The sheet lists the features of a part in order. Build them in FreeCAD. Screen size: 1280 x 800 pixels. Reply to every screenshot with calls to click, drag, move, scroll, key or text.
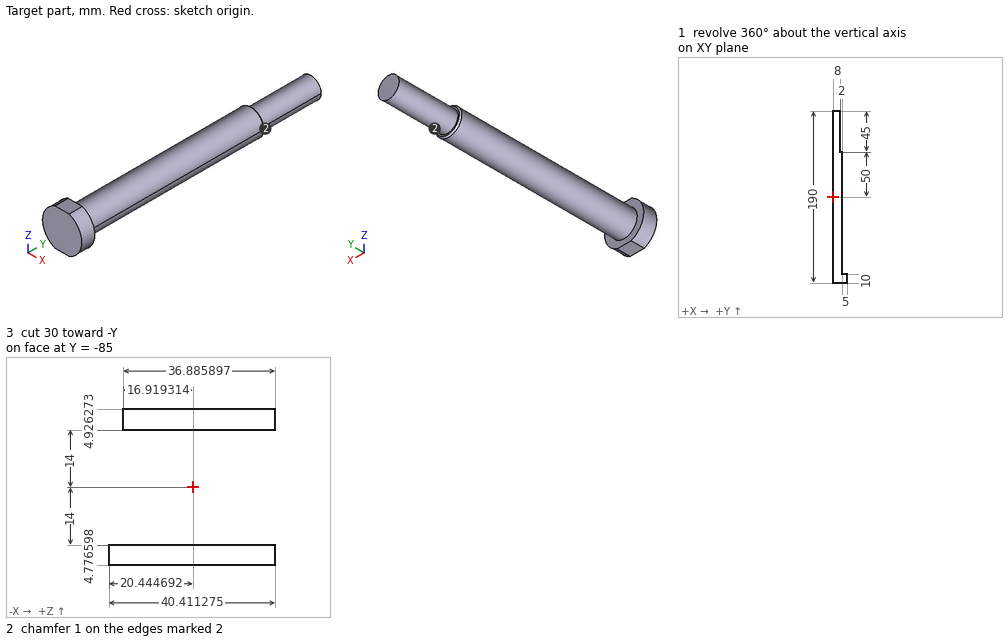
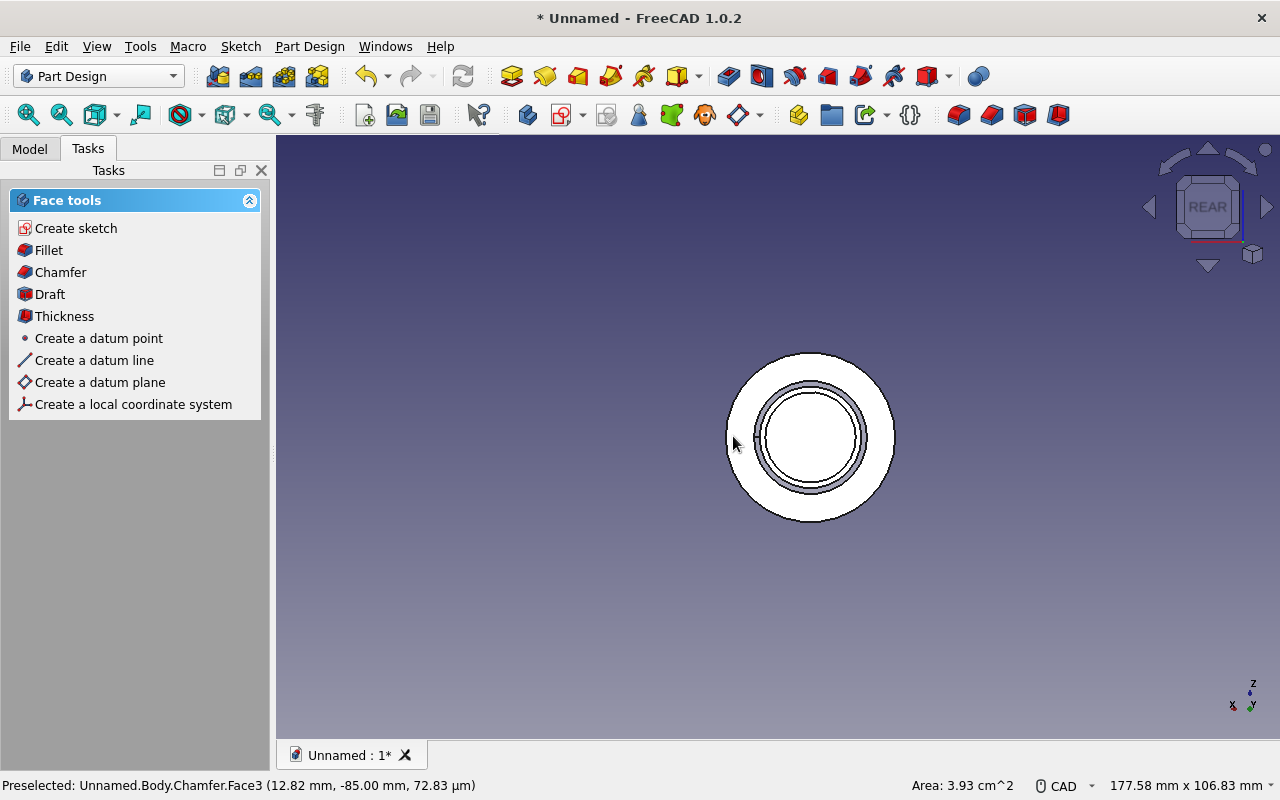
click(560, 116)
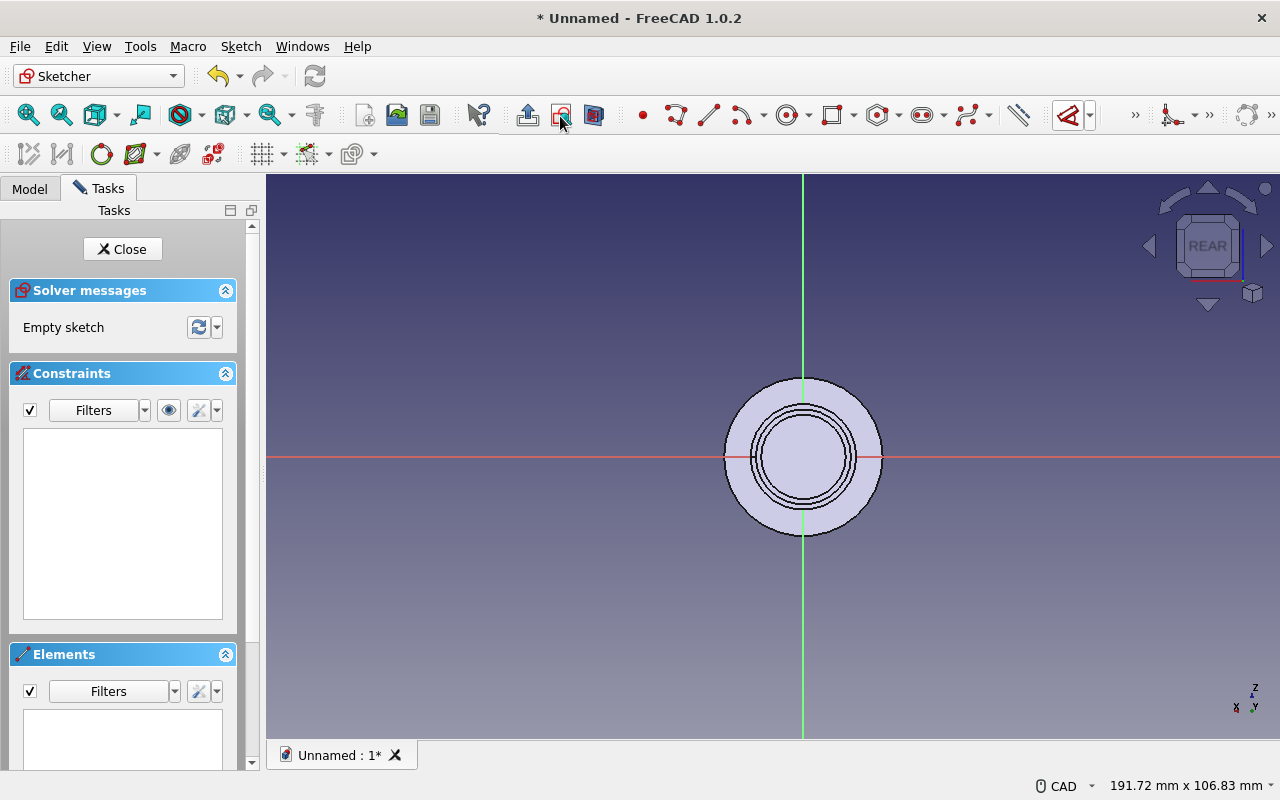
scroll(921, 456, up, 3)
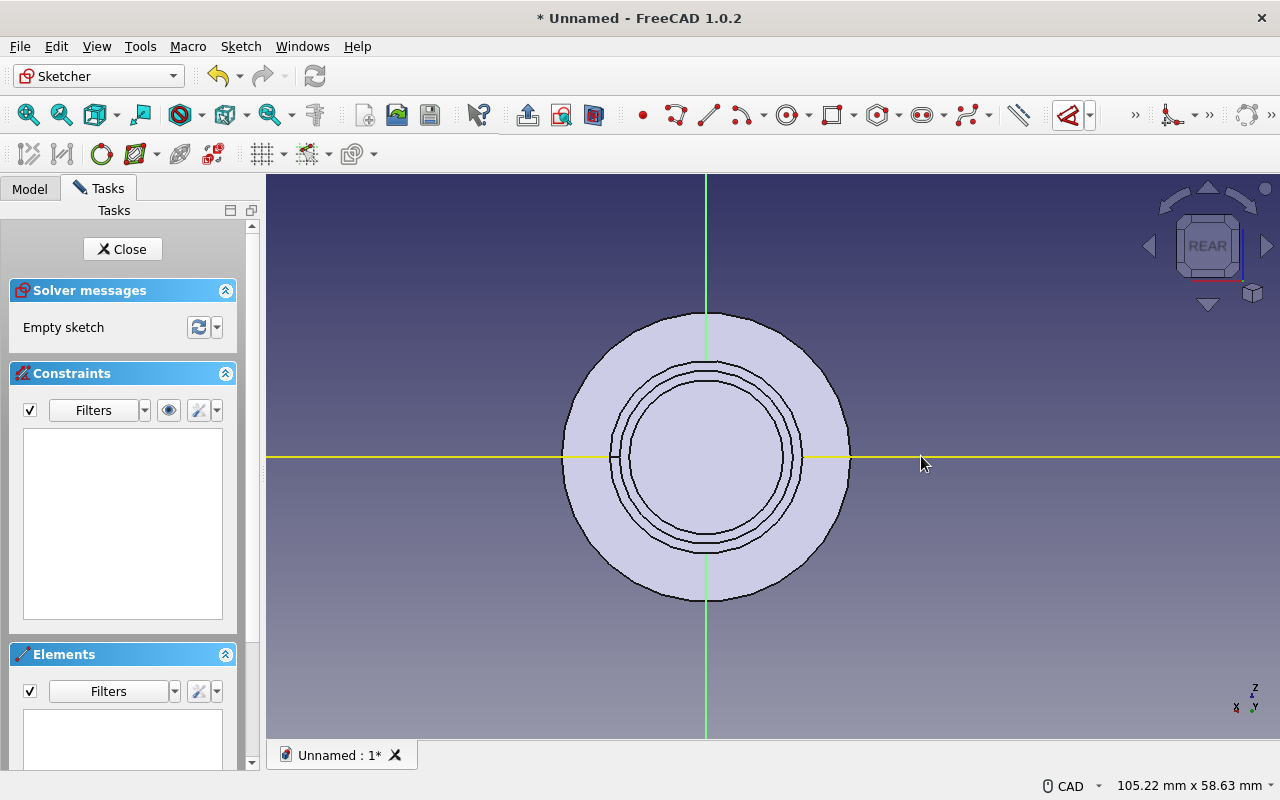
click(832, 116)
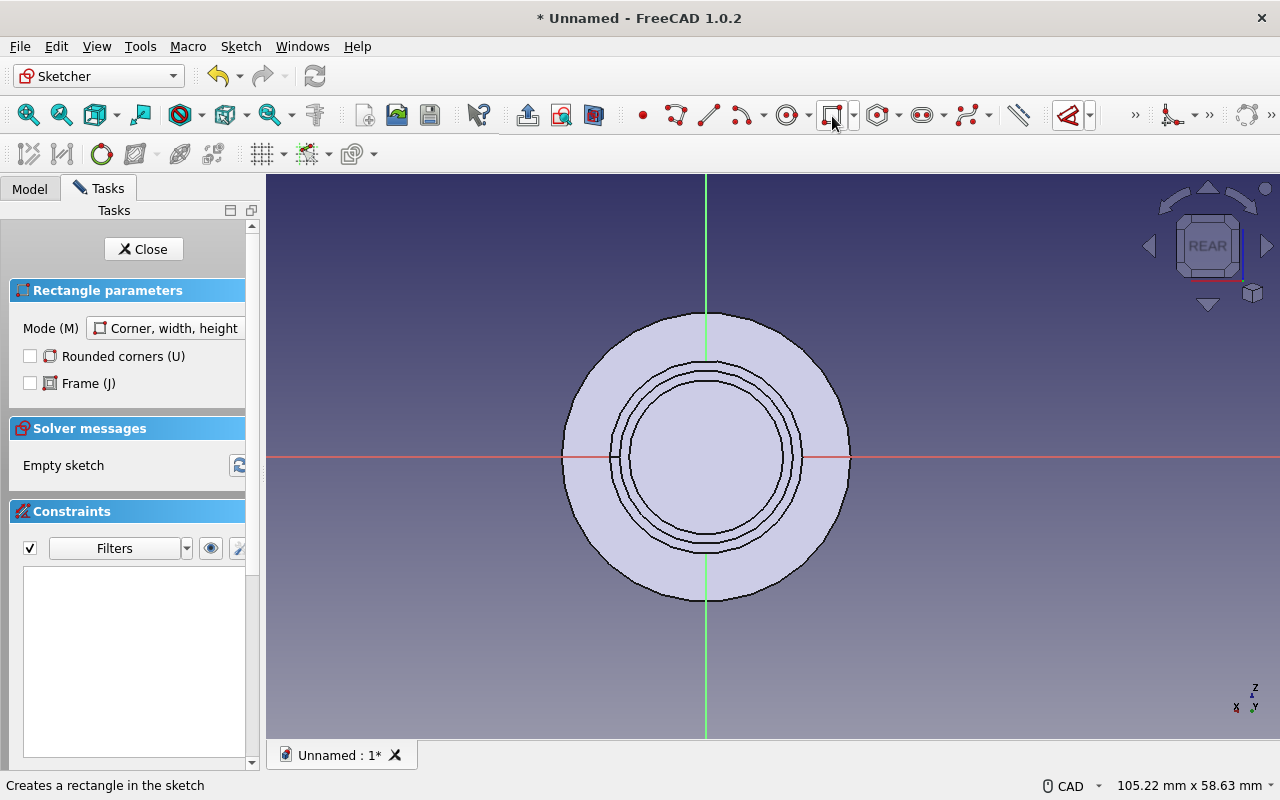
click(543, 275)
click(899, 322)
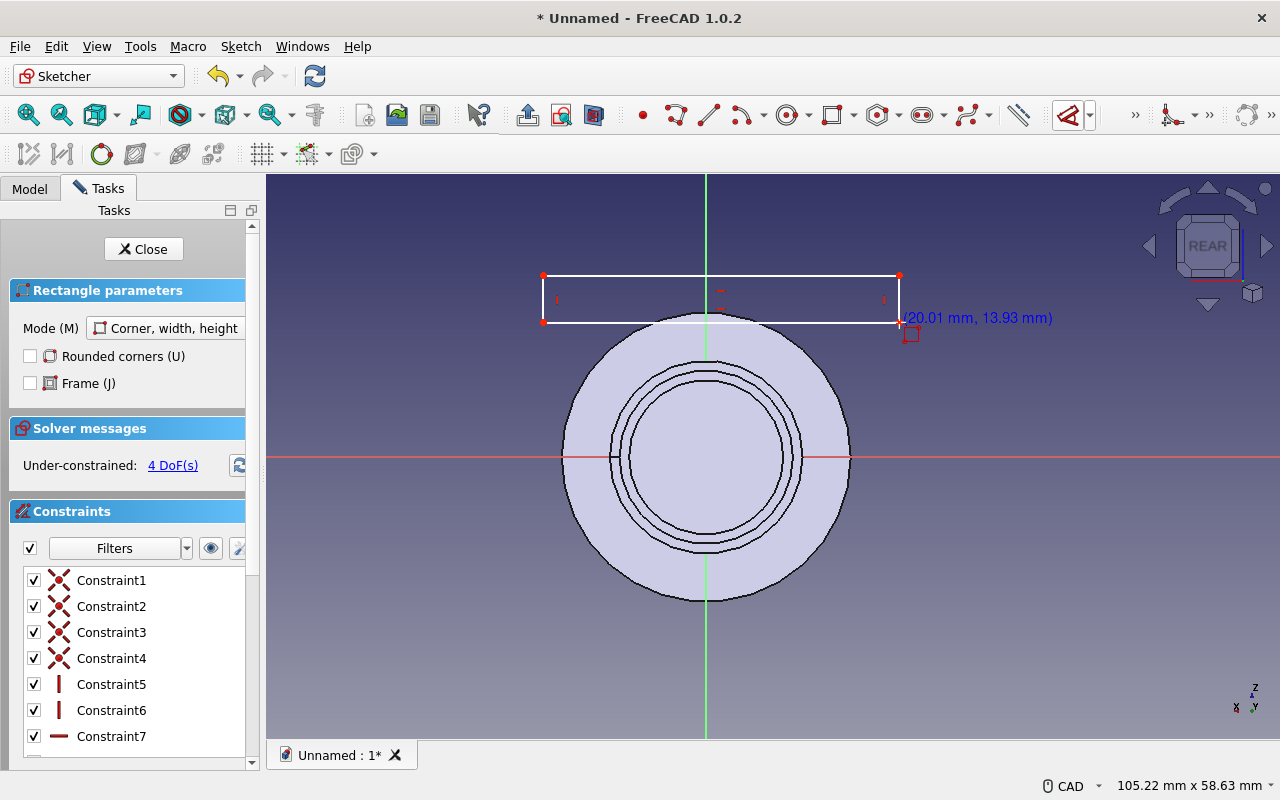
click(509, 592)
click(899, 638)
key(Escape)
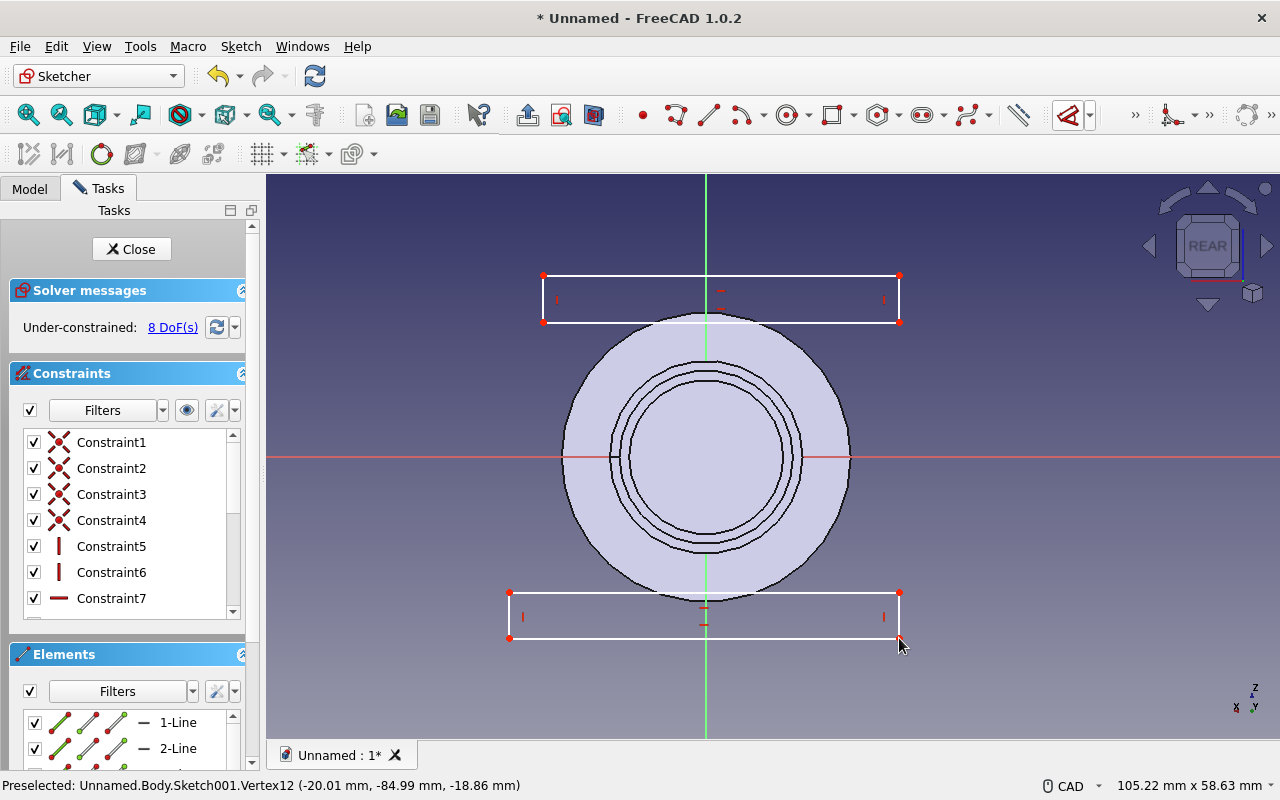
click(543, 323)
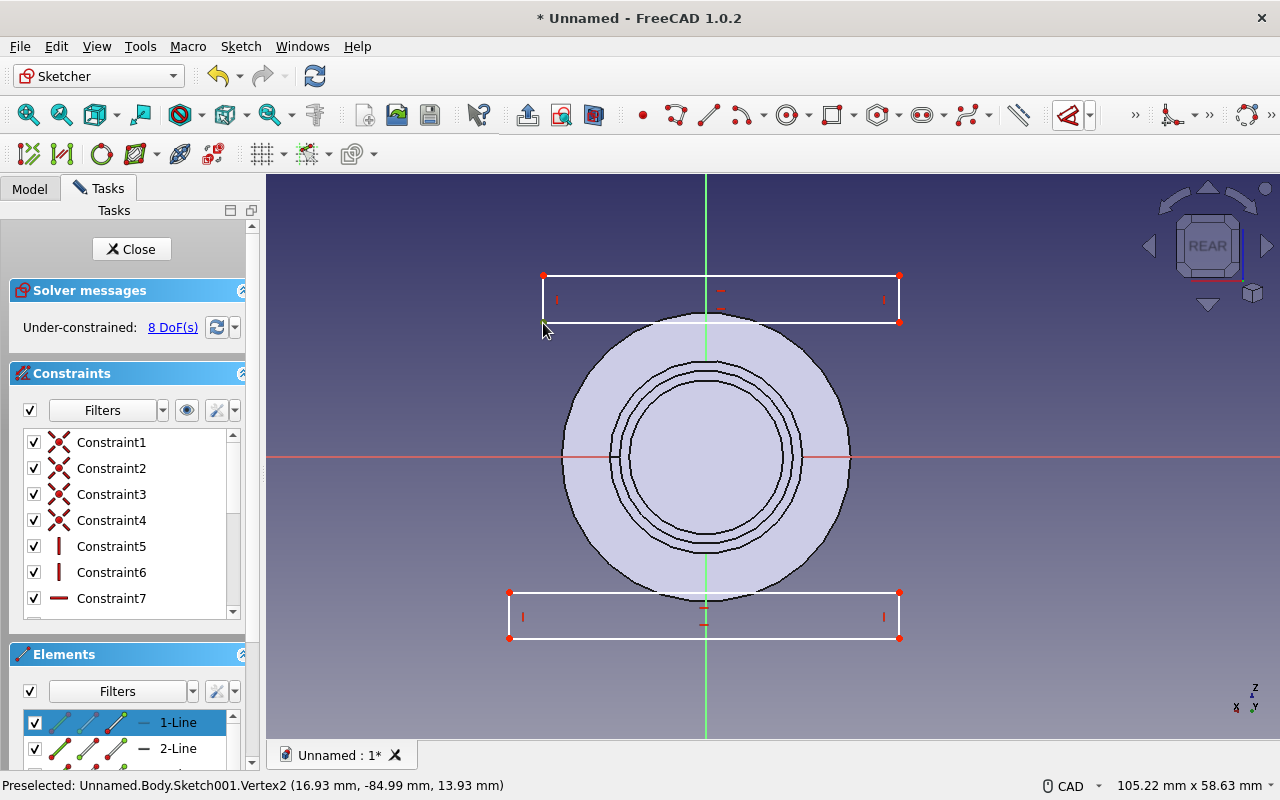
key(i)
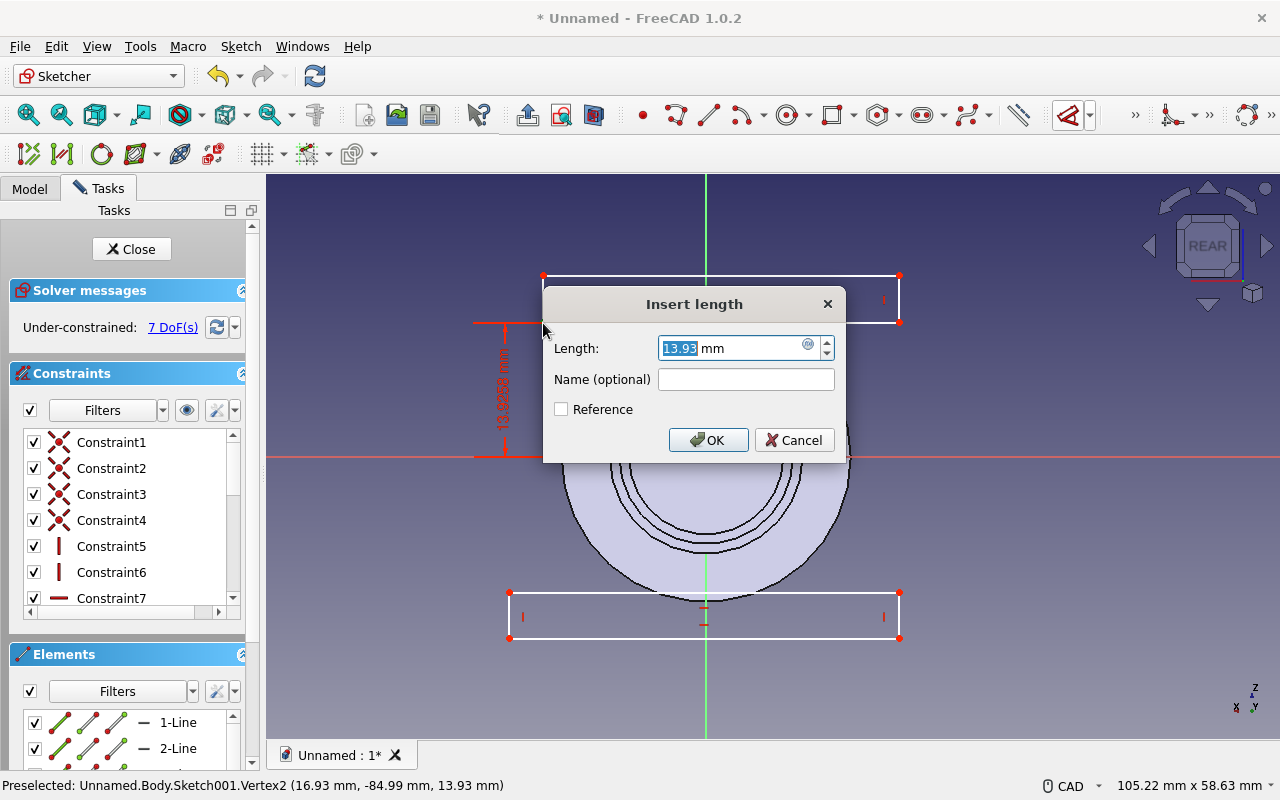
text(14)
key(Return)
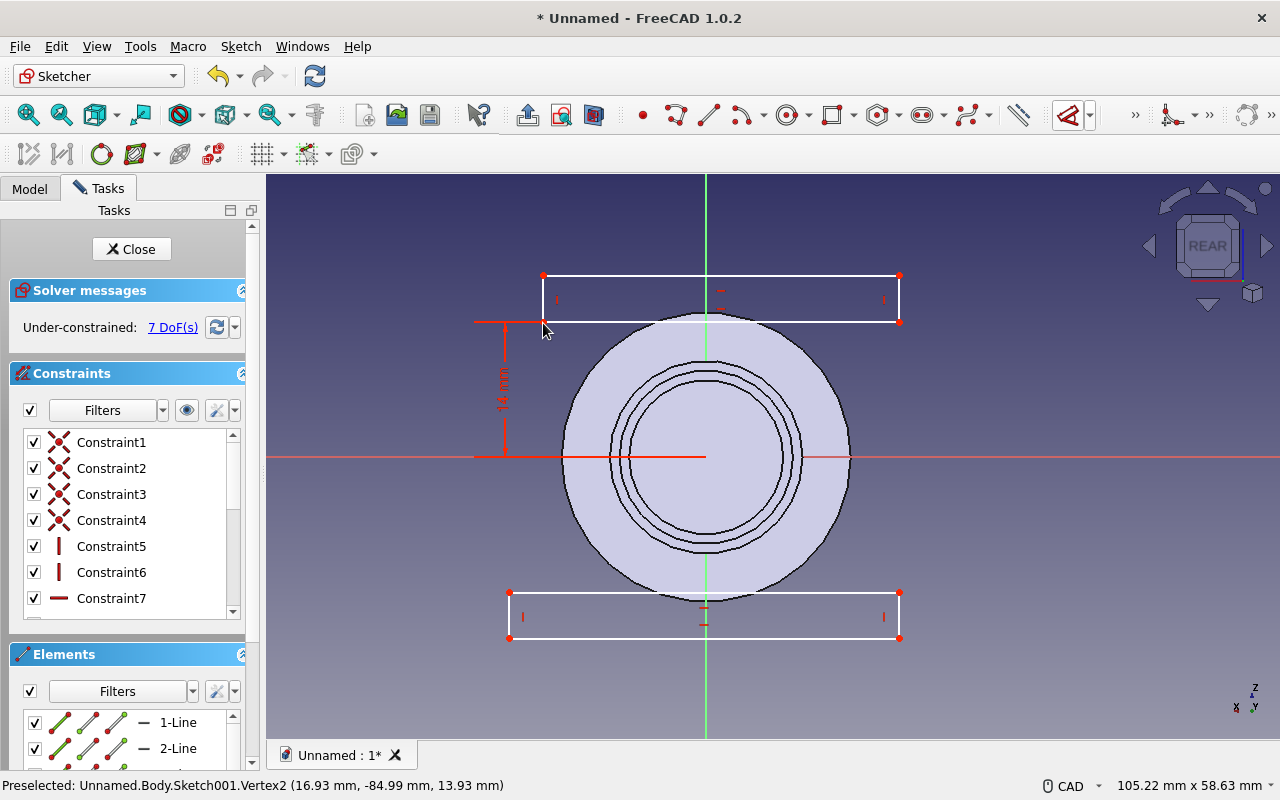
click(509, 593)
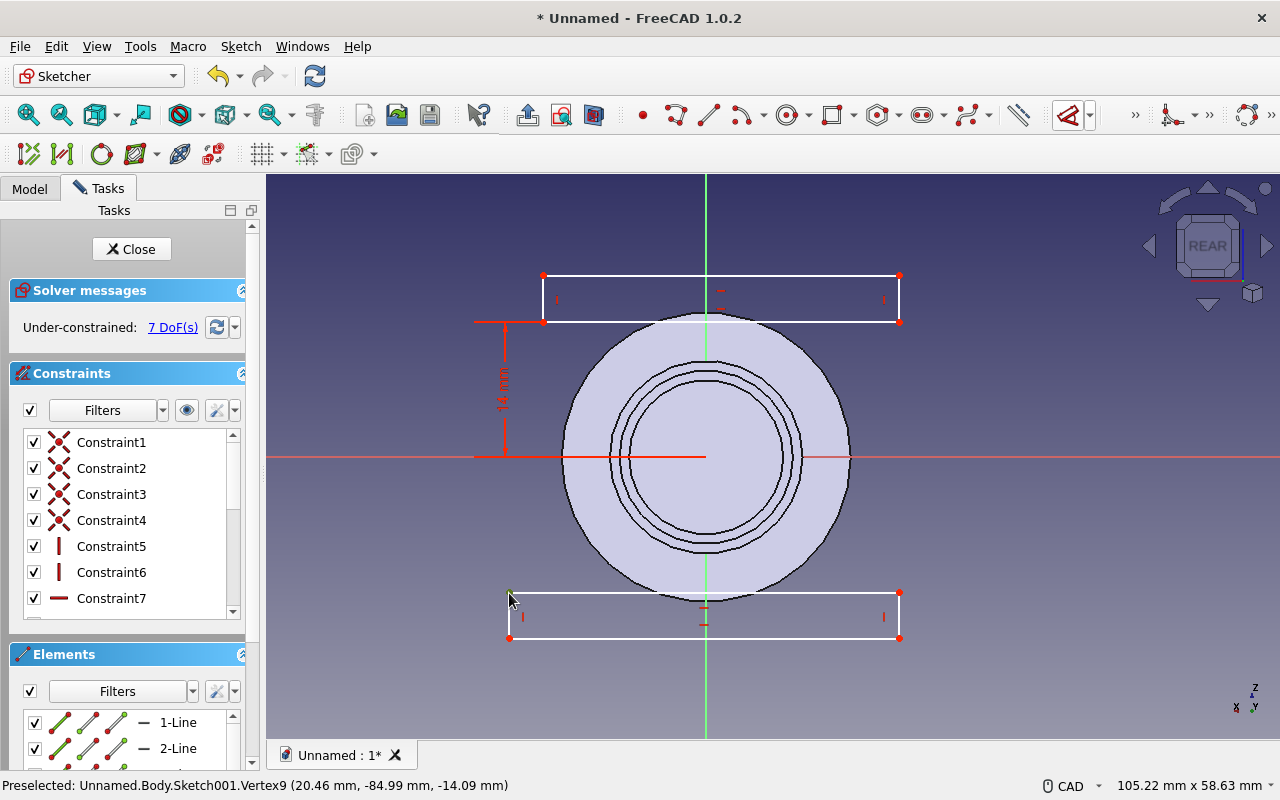
key(i)